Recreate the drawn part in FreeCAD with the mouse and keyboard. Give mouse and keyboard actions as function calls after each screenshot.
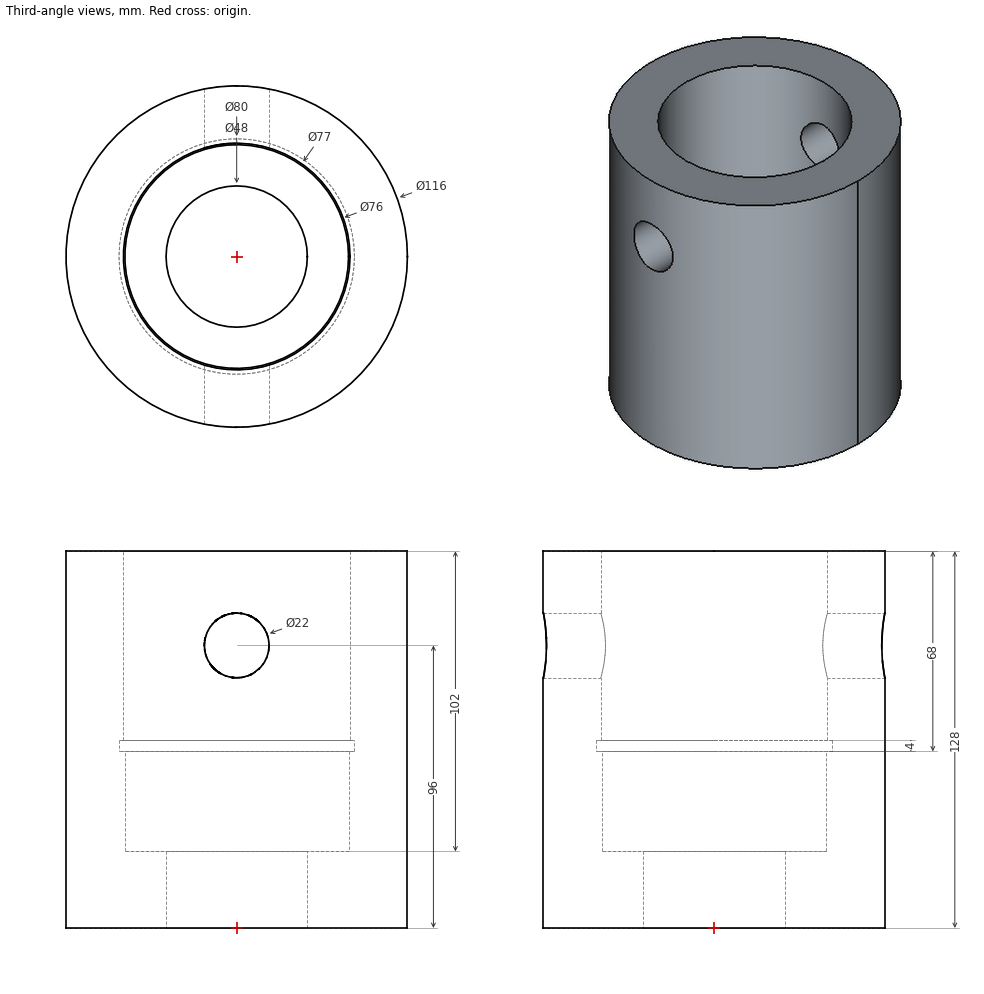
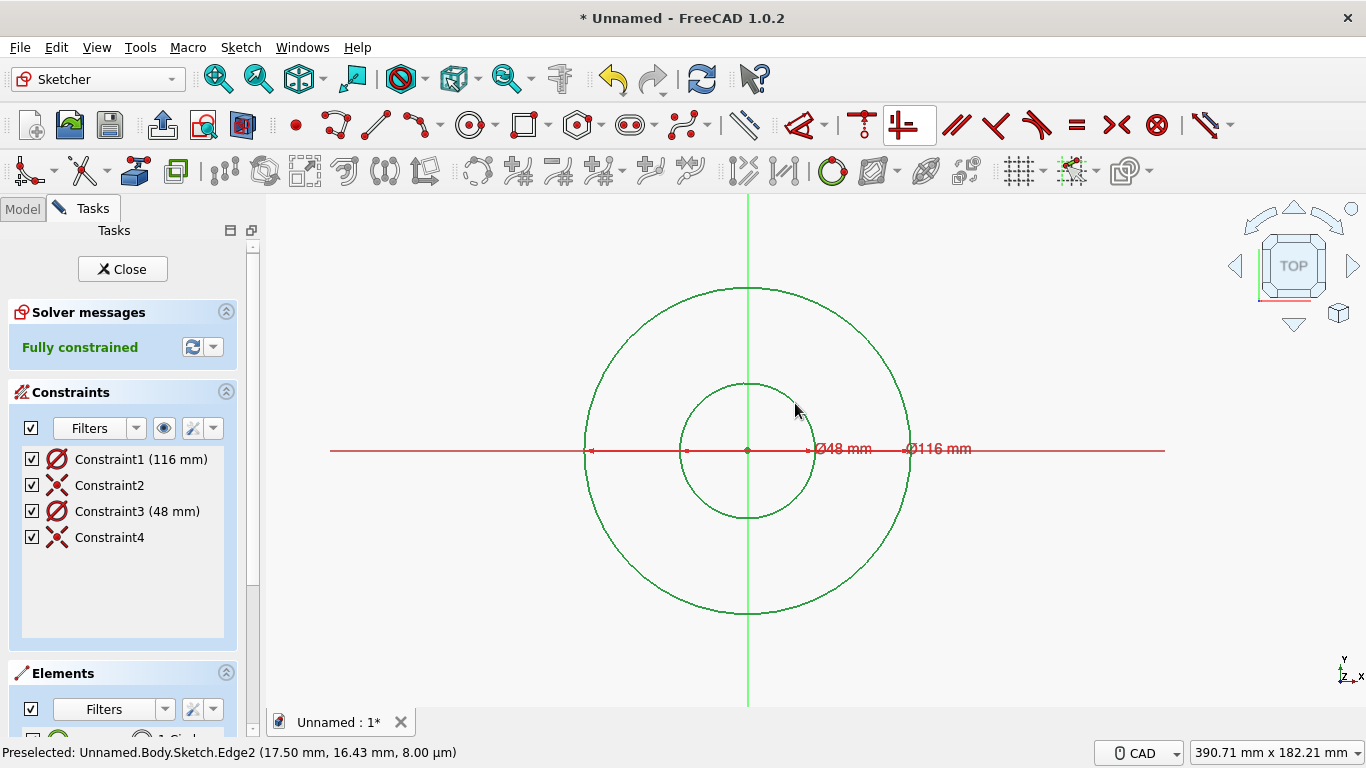
click(123, 269)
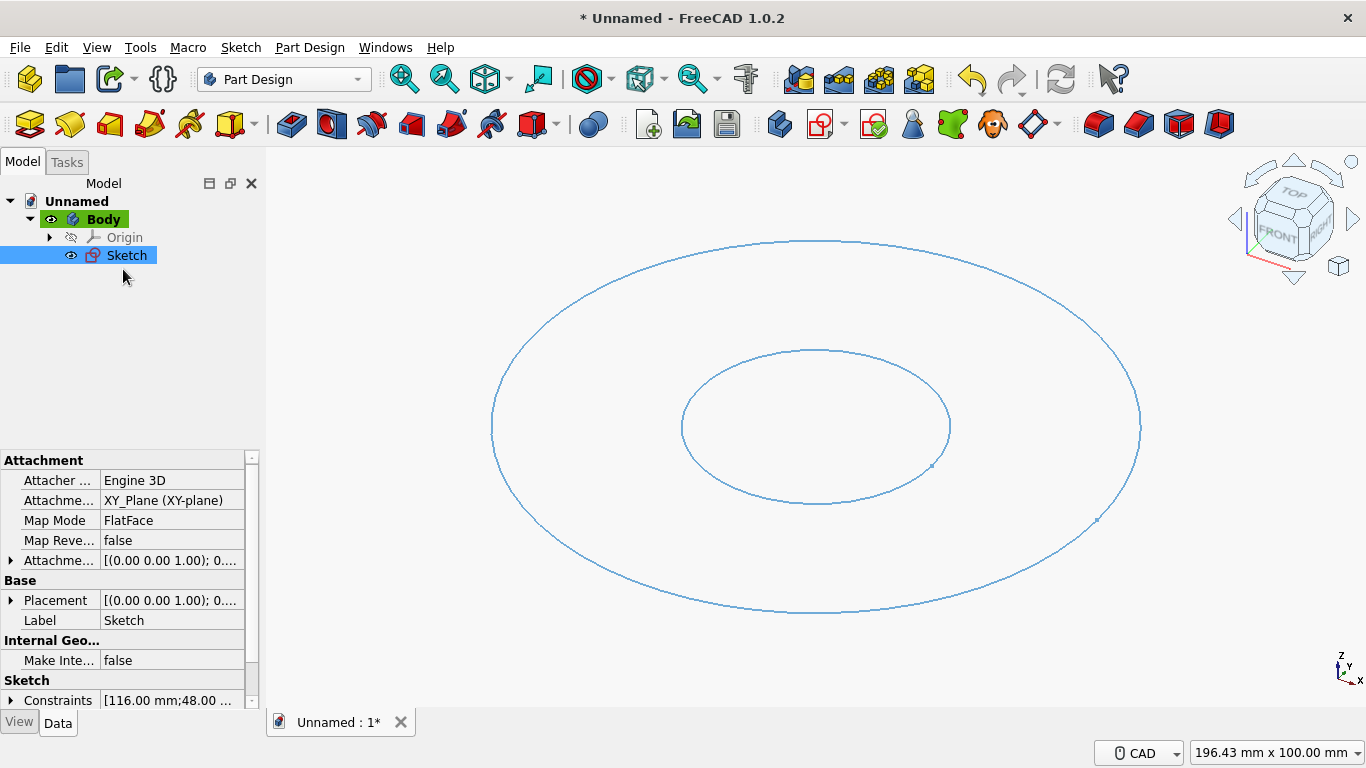
click(30, 124)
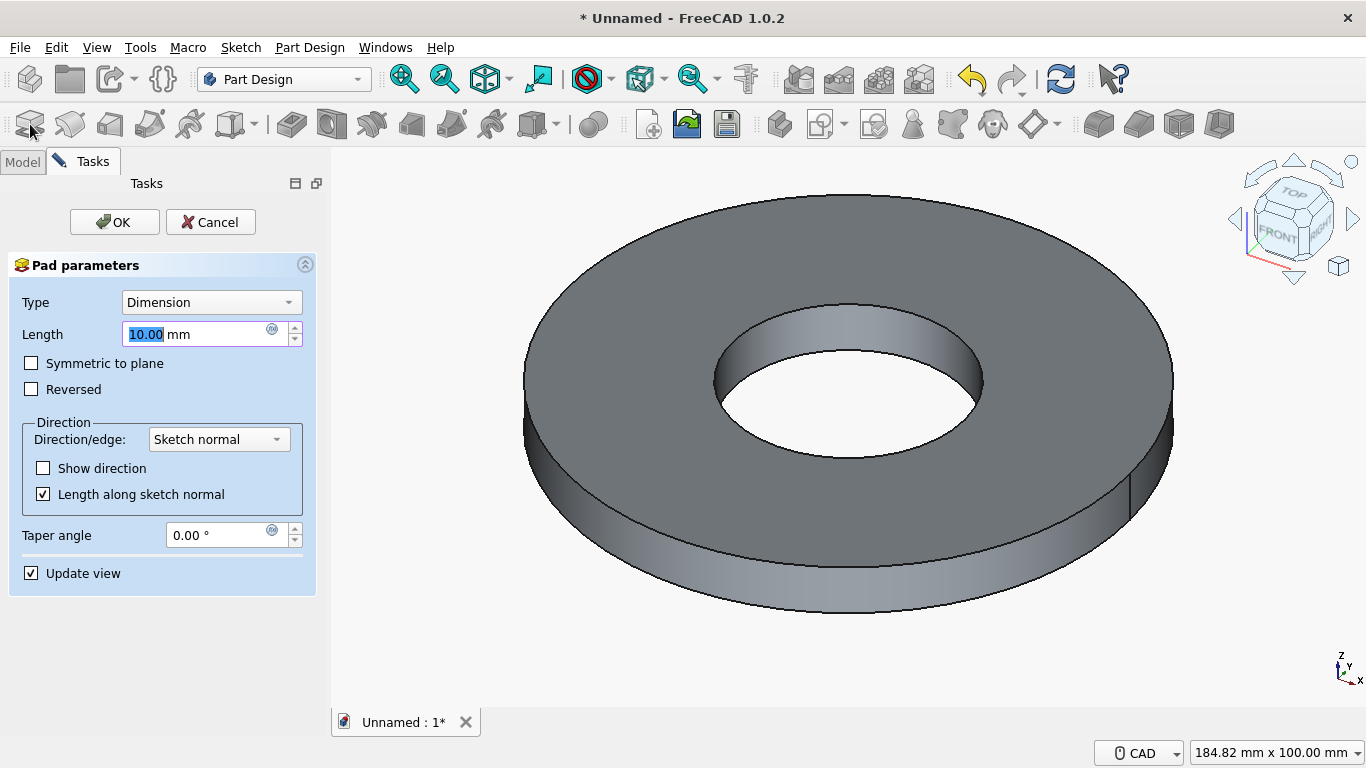
text(128)
key(Tab)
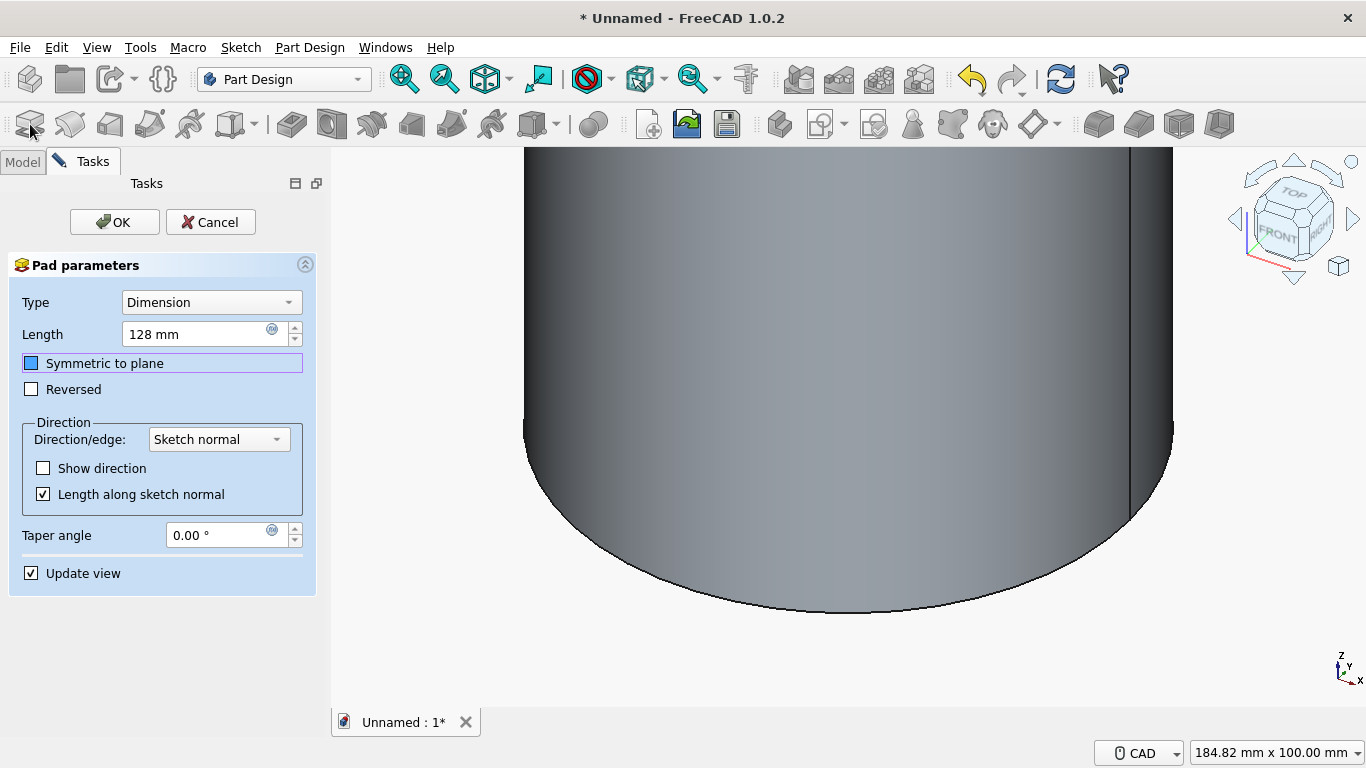
click(115, 222)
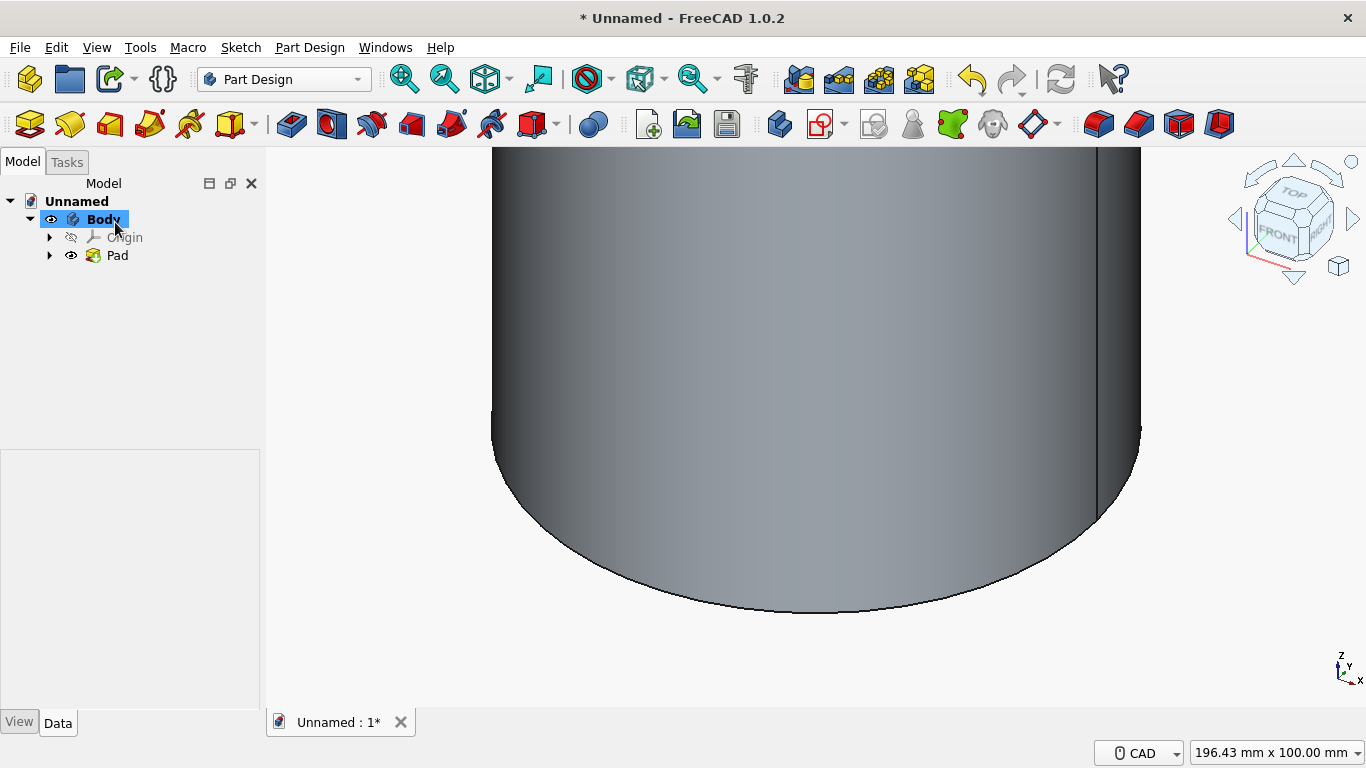
key(v)
key(f)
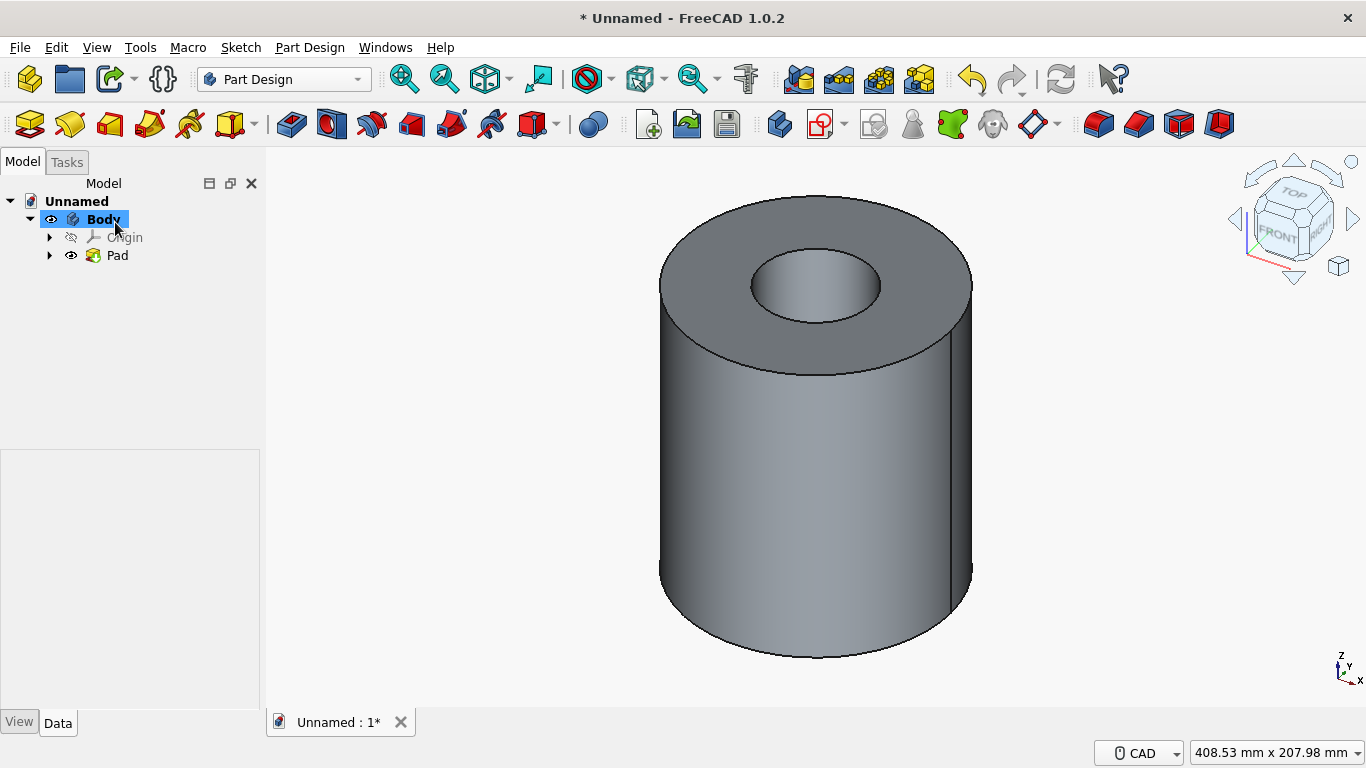
click(915, 288)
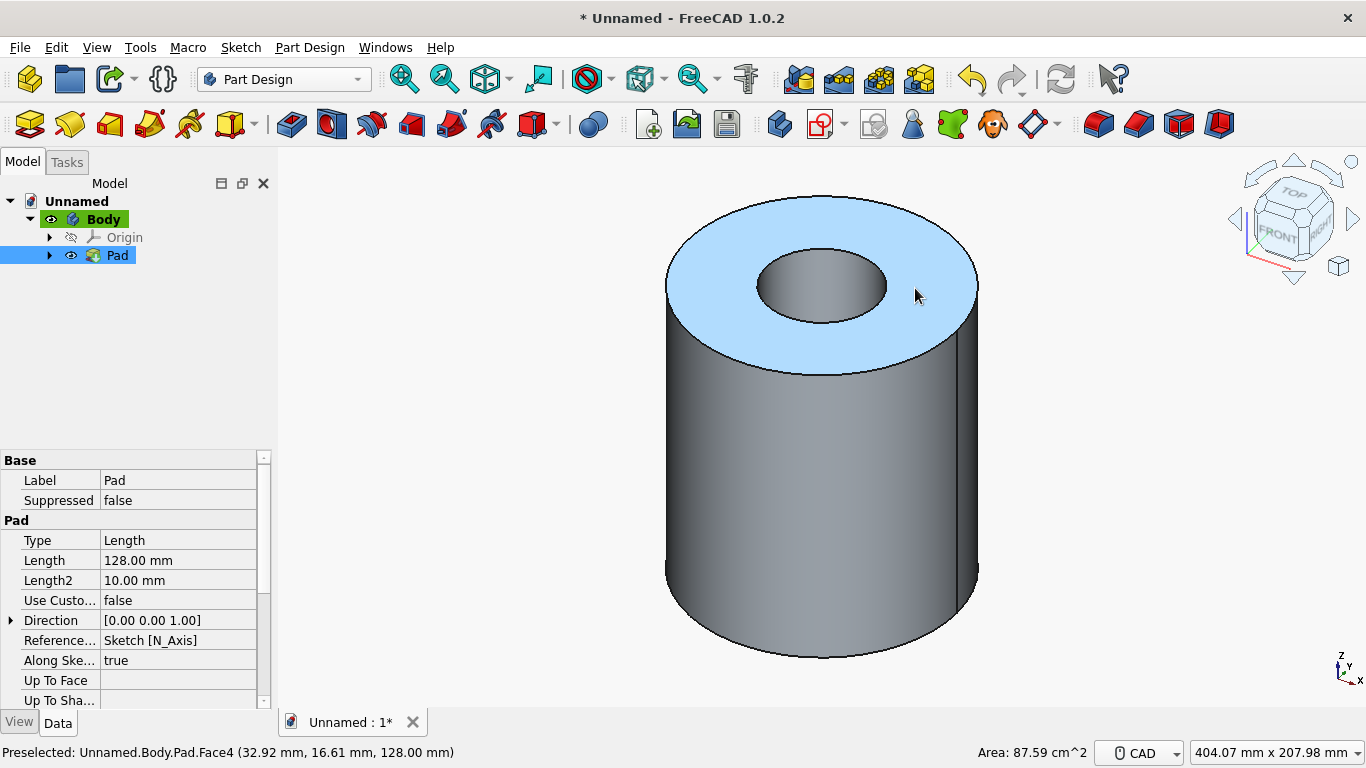
click(820, 124)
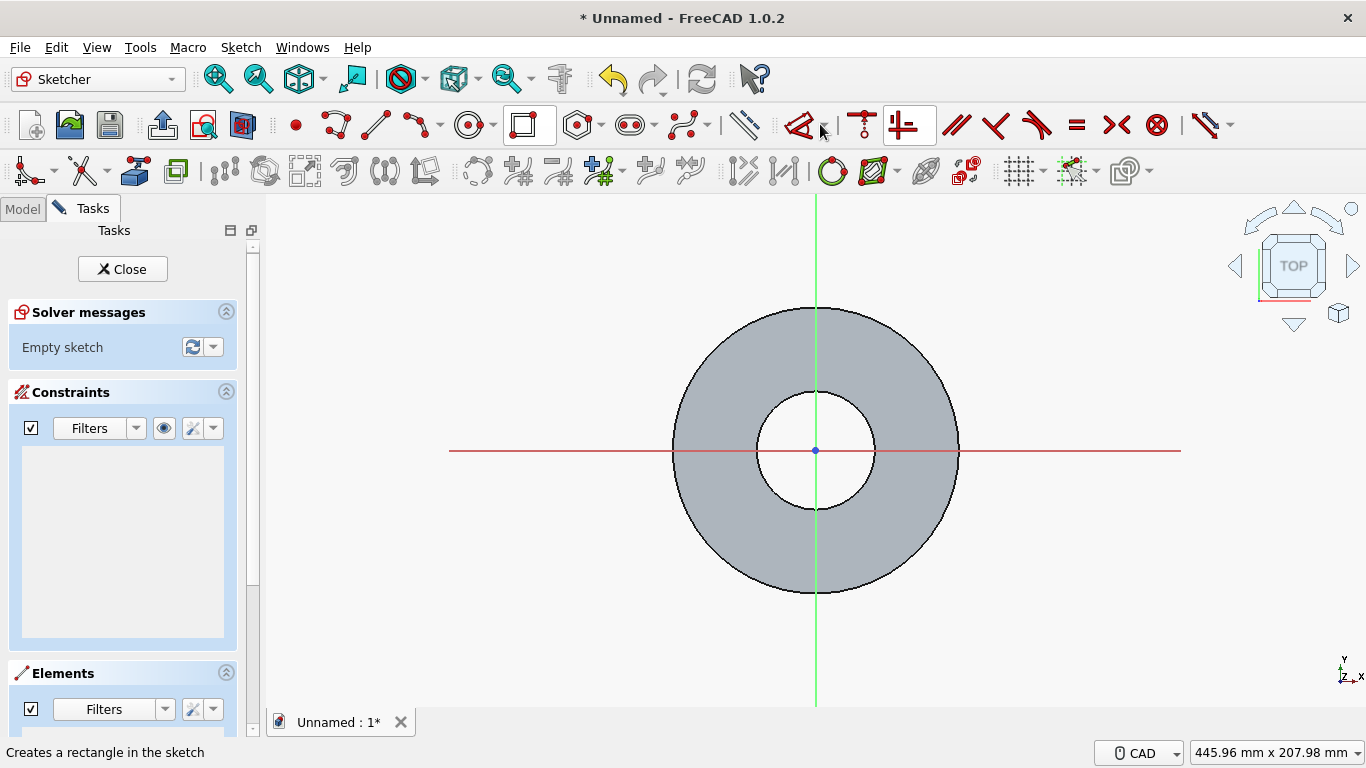
scroll(899, 450, up, 3)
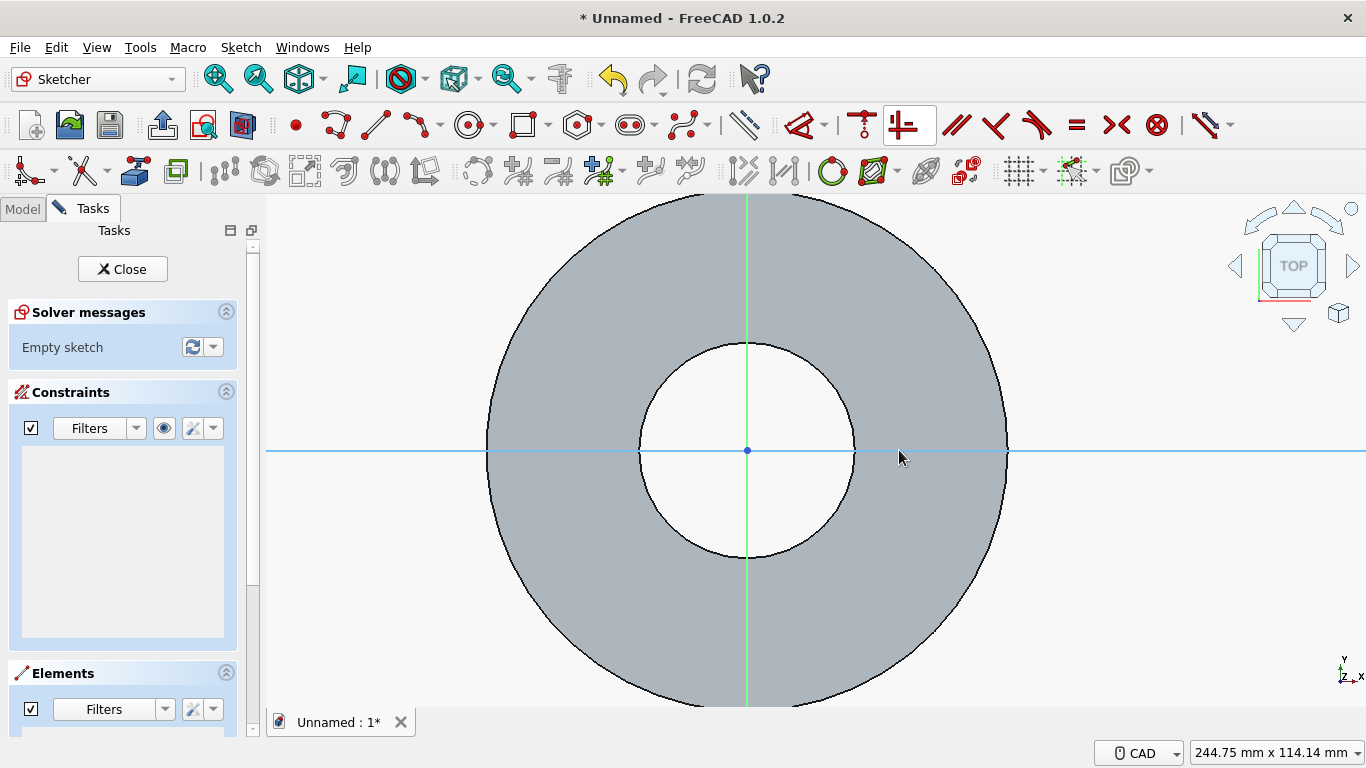
key(g)
key(c)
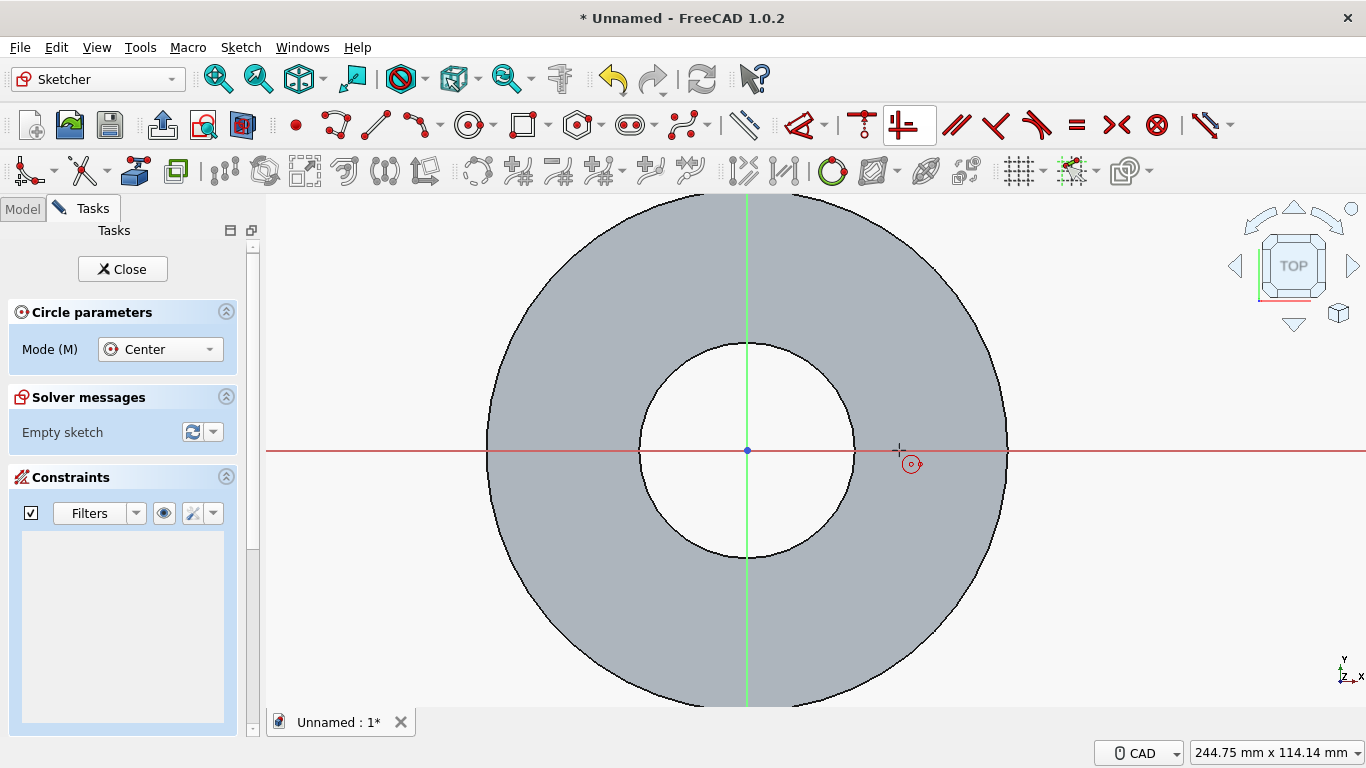
click(747, 450)
move(868, 330)